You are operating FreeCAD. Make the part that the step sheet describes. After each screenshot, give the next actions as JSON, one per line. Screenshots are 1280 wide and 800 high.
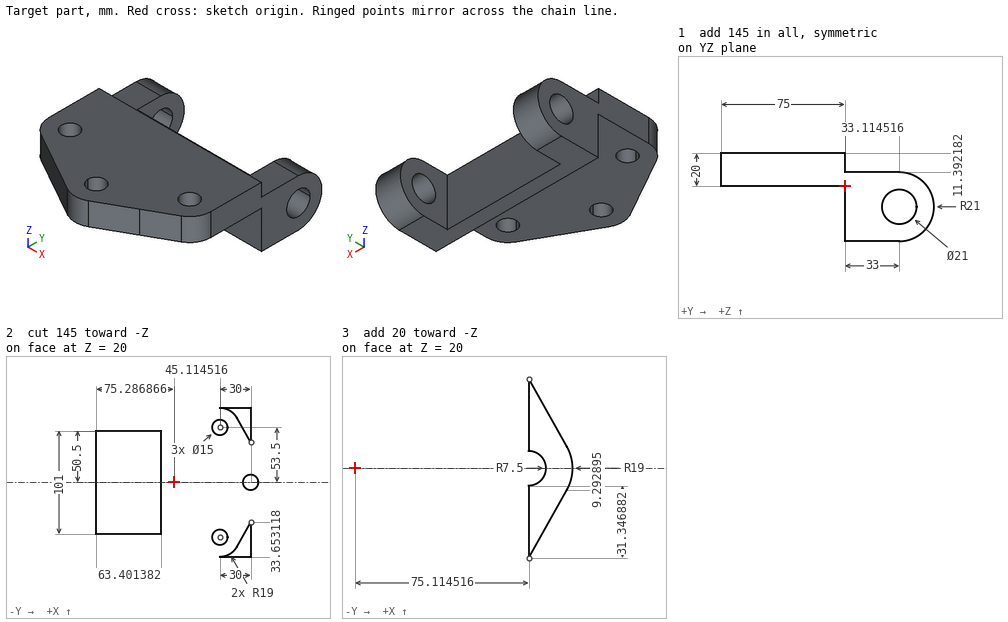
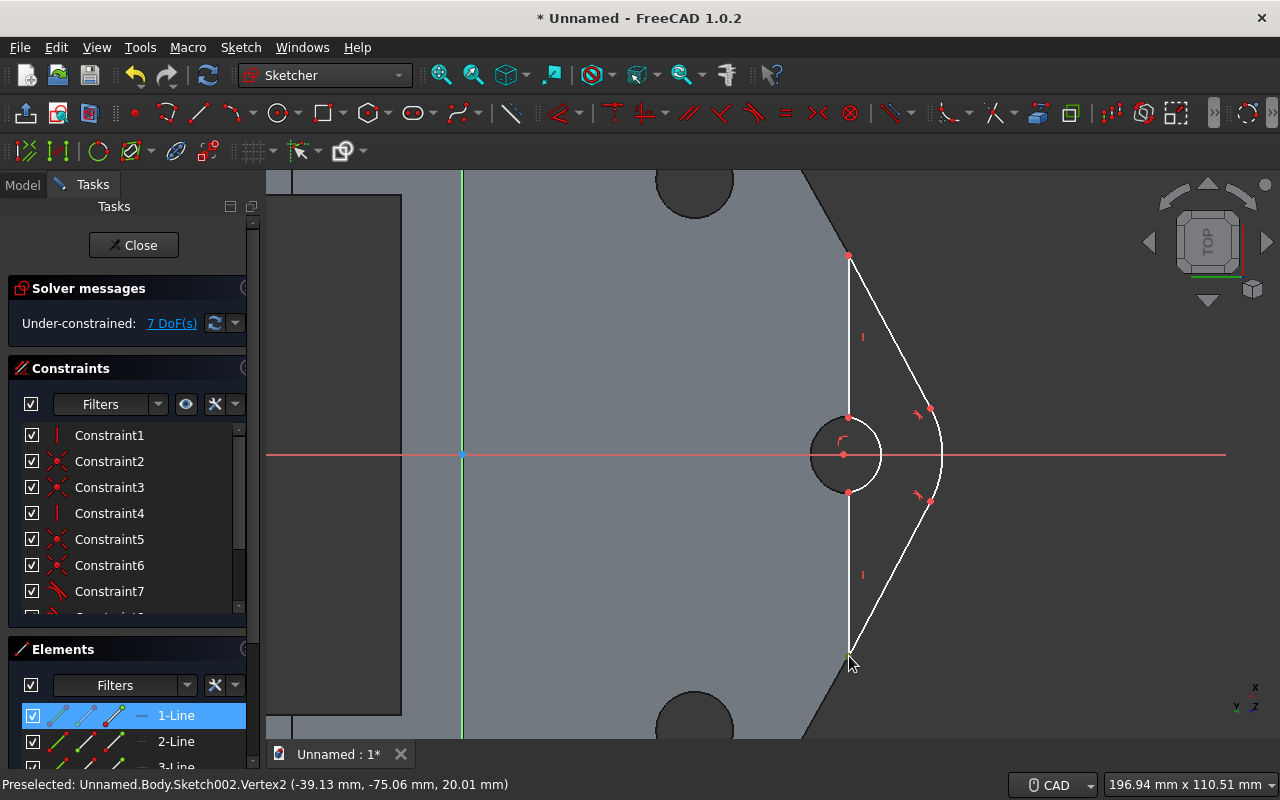
{"action": "left_click", "coordinate": [849, 255]}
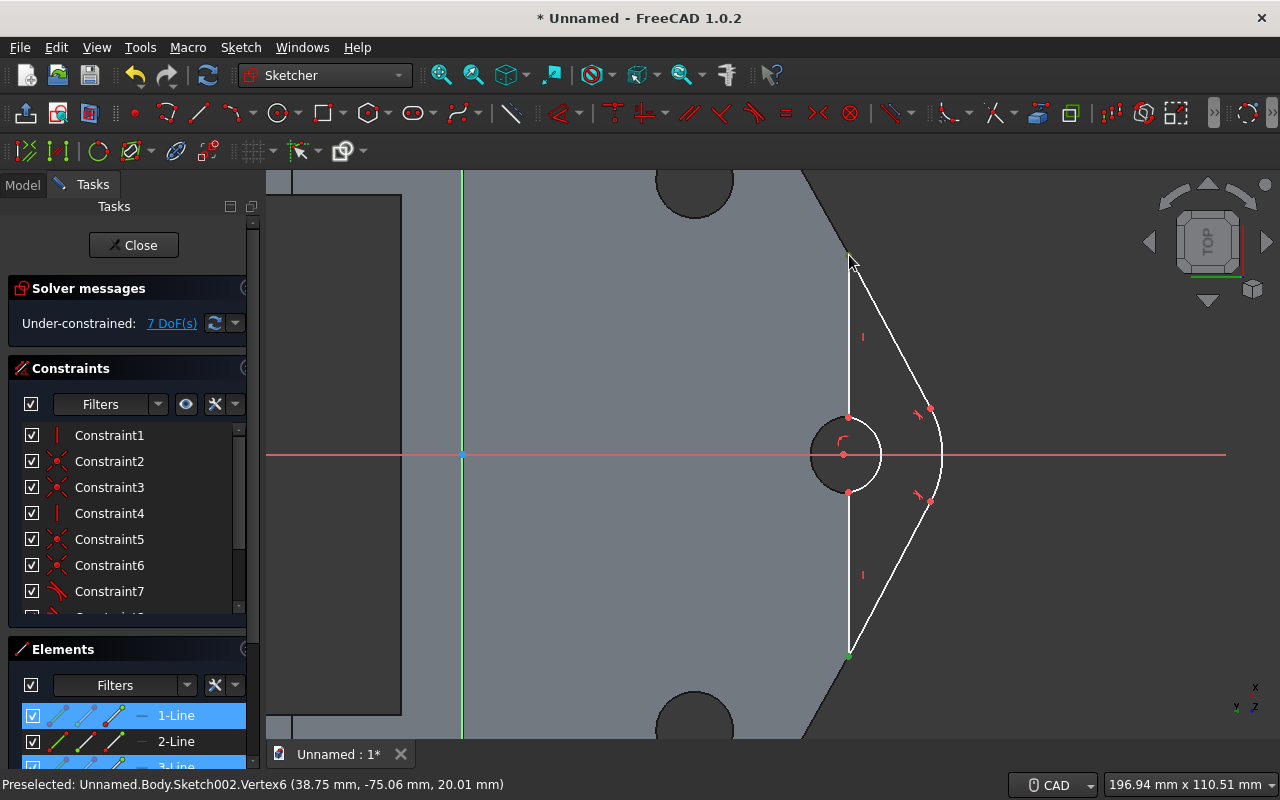
{"action": "left_click", "coordinate": [353, 455]}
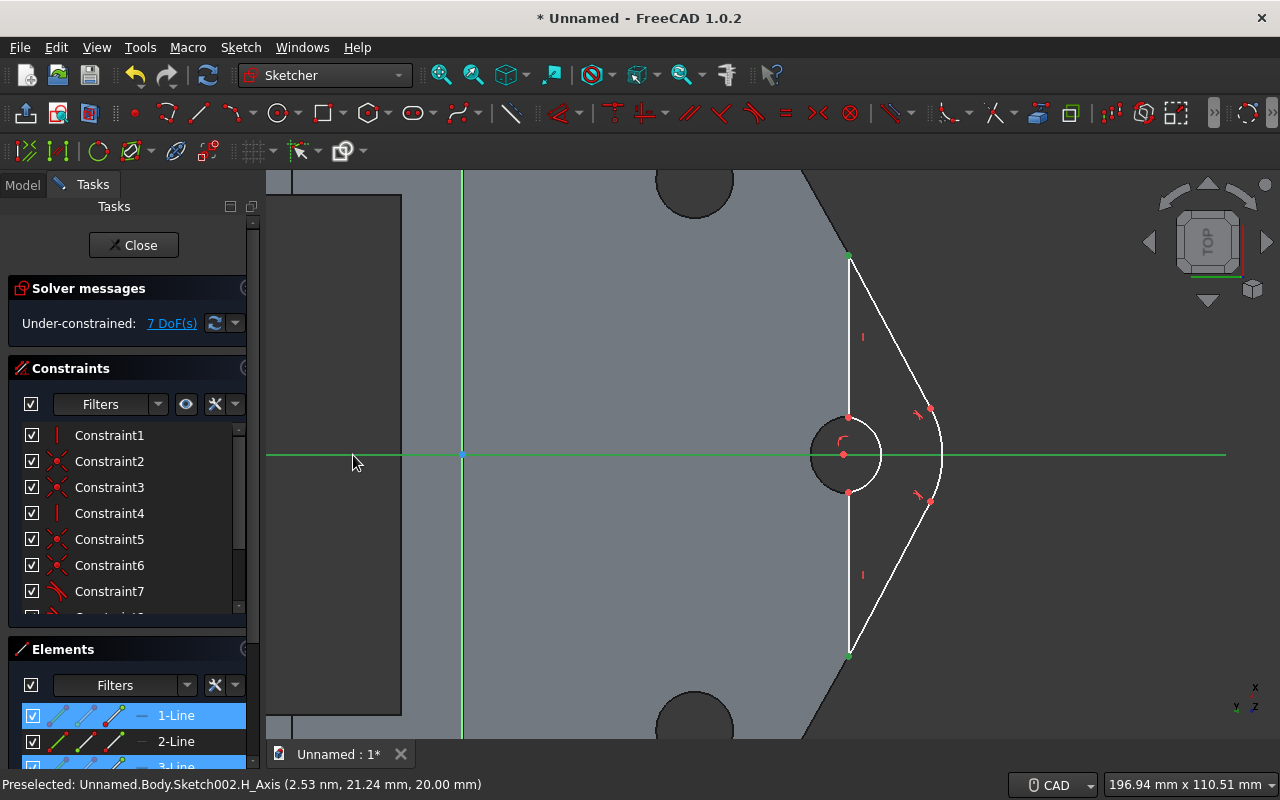
{"action": "left_click", "coordinate": [818, 114]}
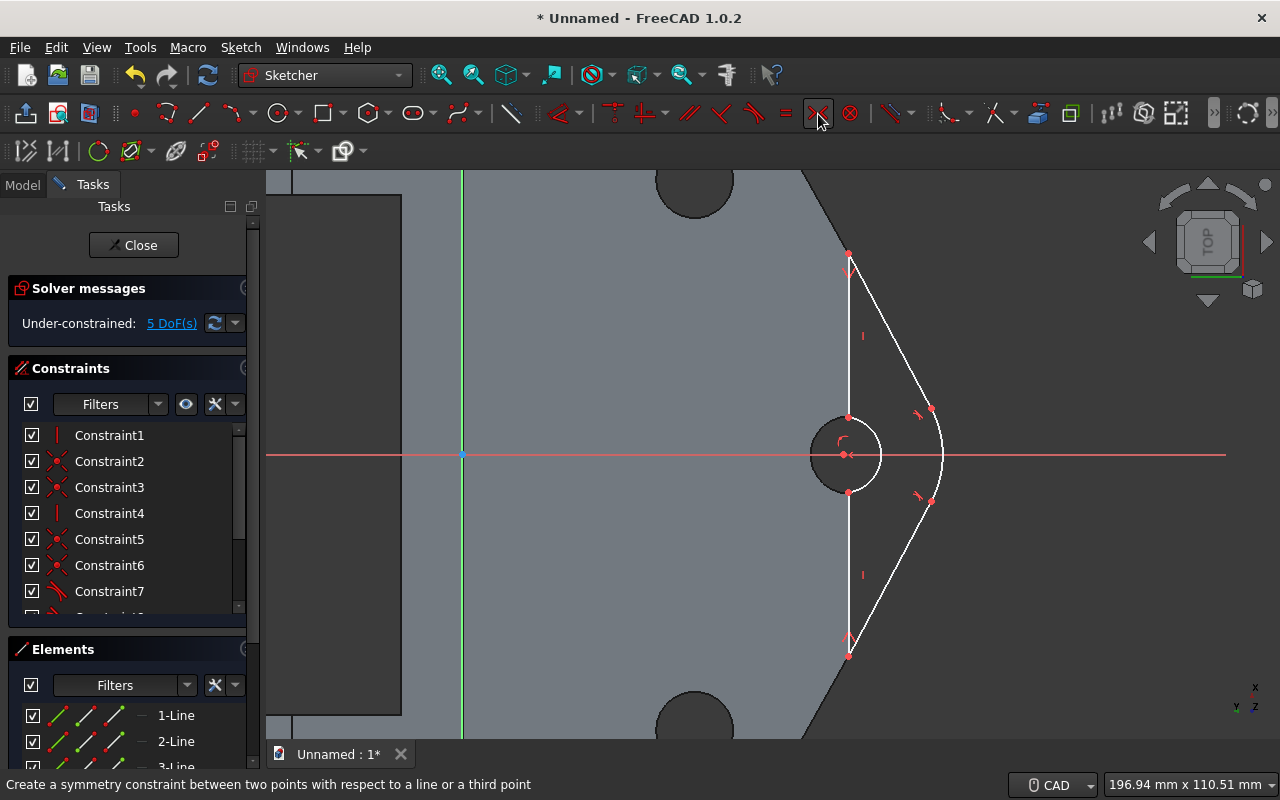
{"action": "left_click", "coordinate": [558, 114]}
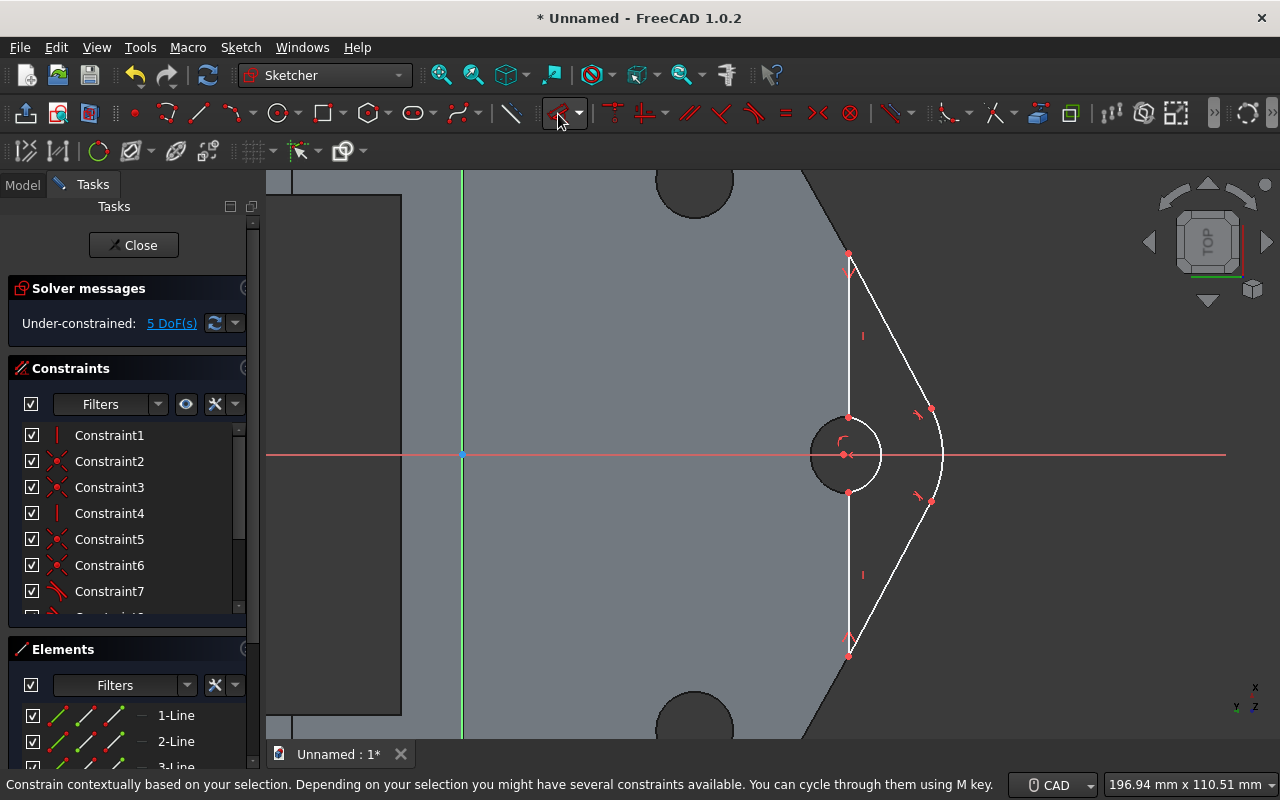
{"action": "left_click", "coordinate": [941, 474]}
{"action": "left_click", "coordinate": [972, 480]}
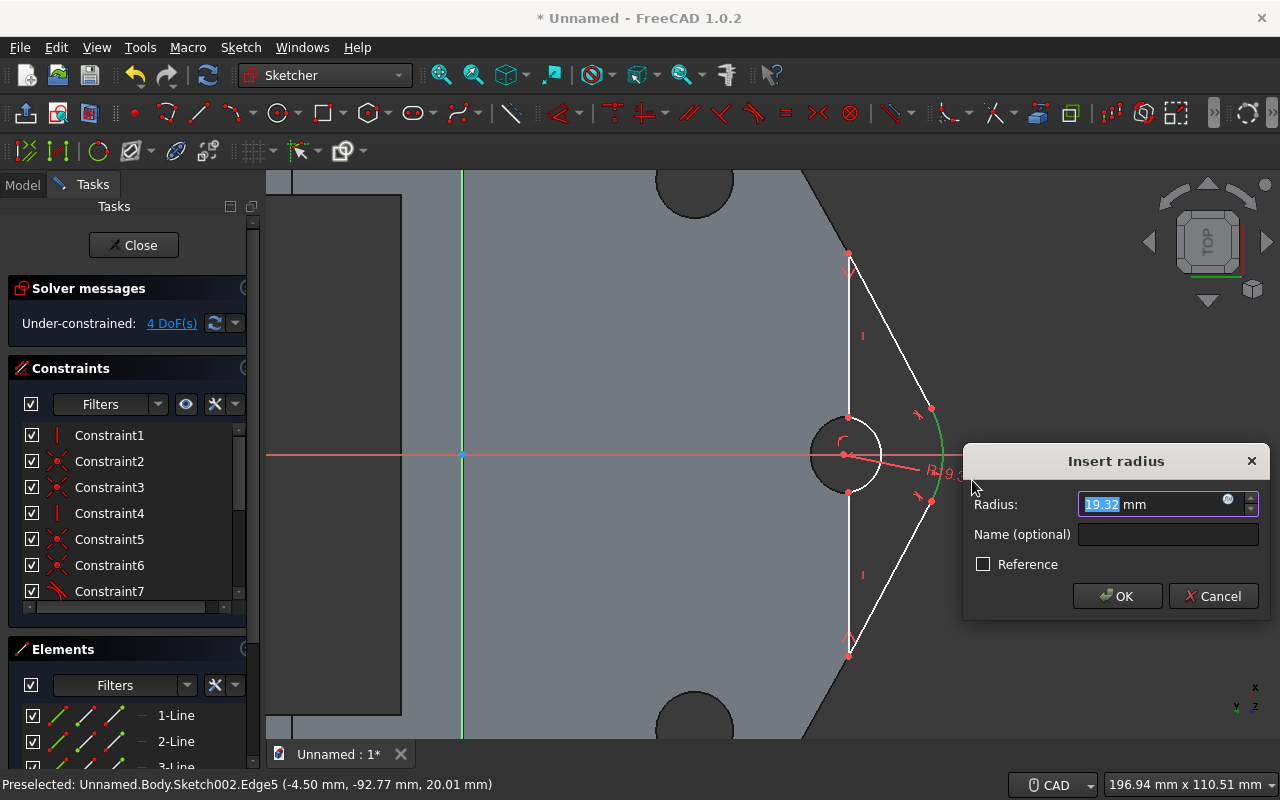
{"action": "type", "text": "19"}
{"action": "key", "text": "Return"}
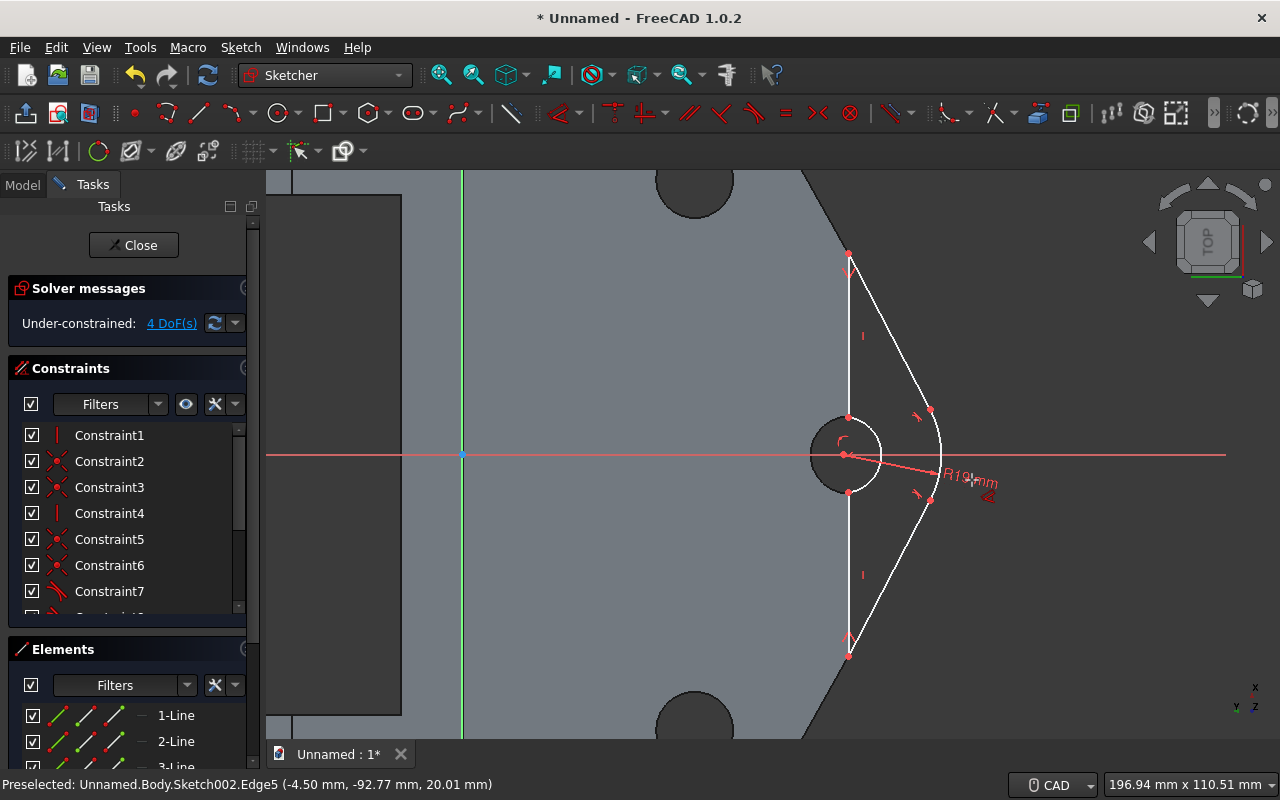
{"action": "left_click", "coordinate": [875, 475]}
{"action": "left_click", "coordinate": [902, 492]}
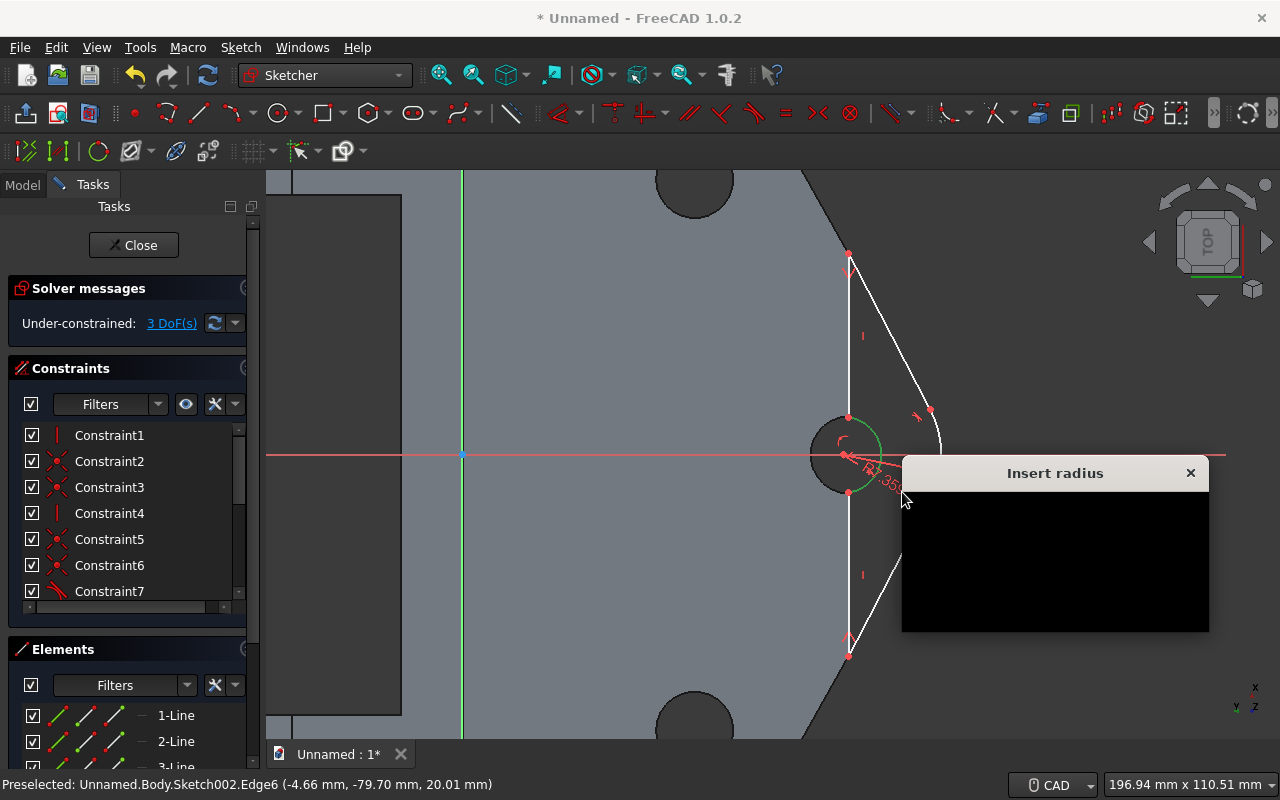
{"action": "type", "text": "7.5"}
{"action": "key", "text": "Return"}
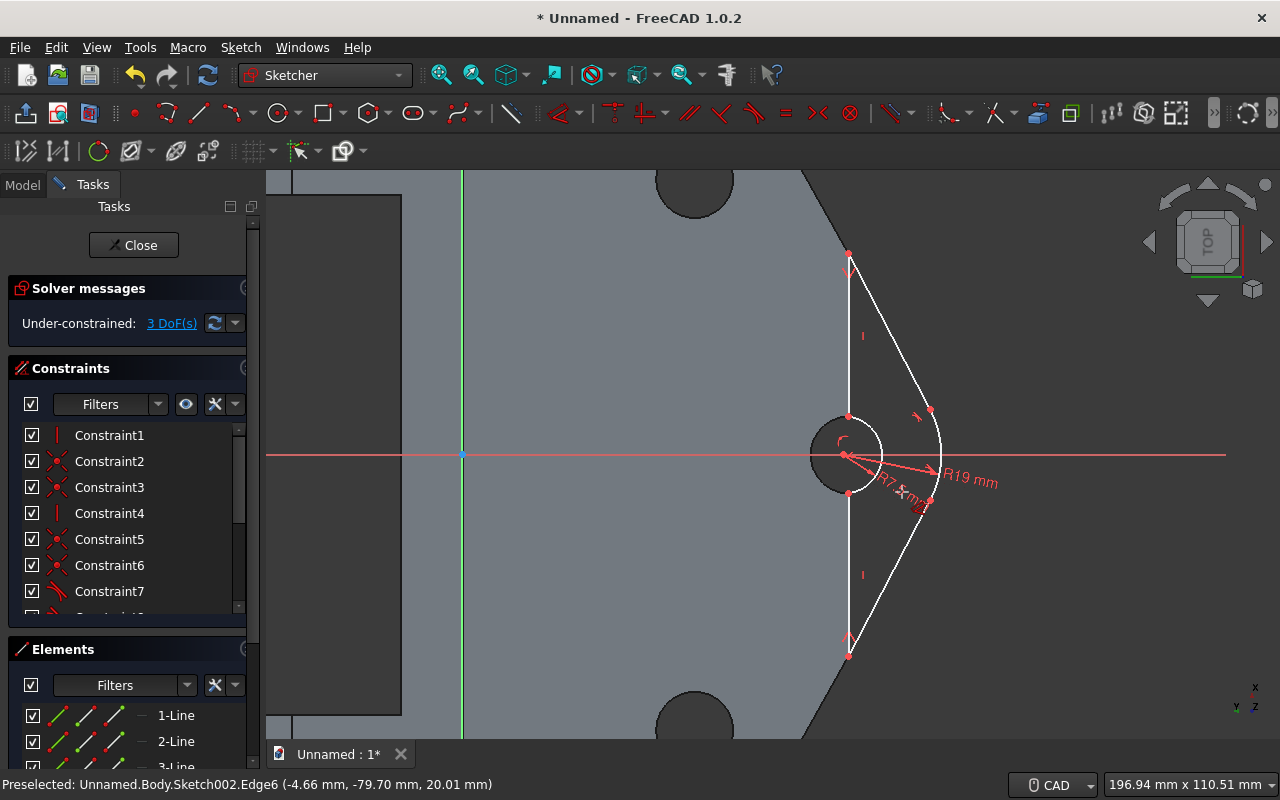
{"action": "left_click", "coordinate": [849, 542]}
{"action": "left_click", "coordinate": [883, 537]}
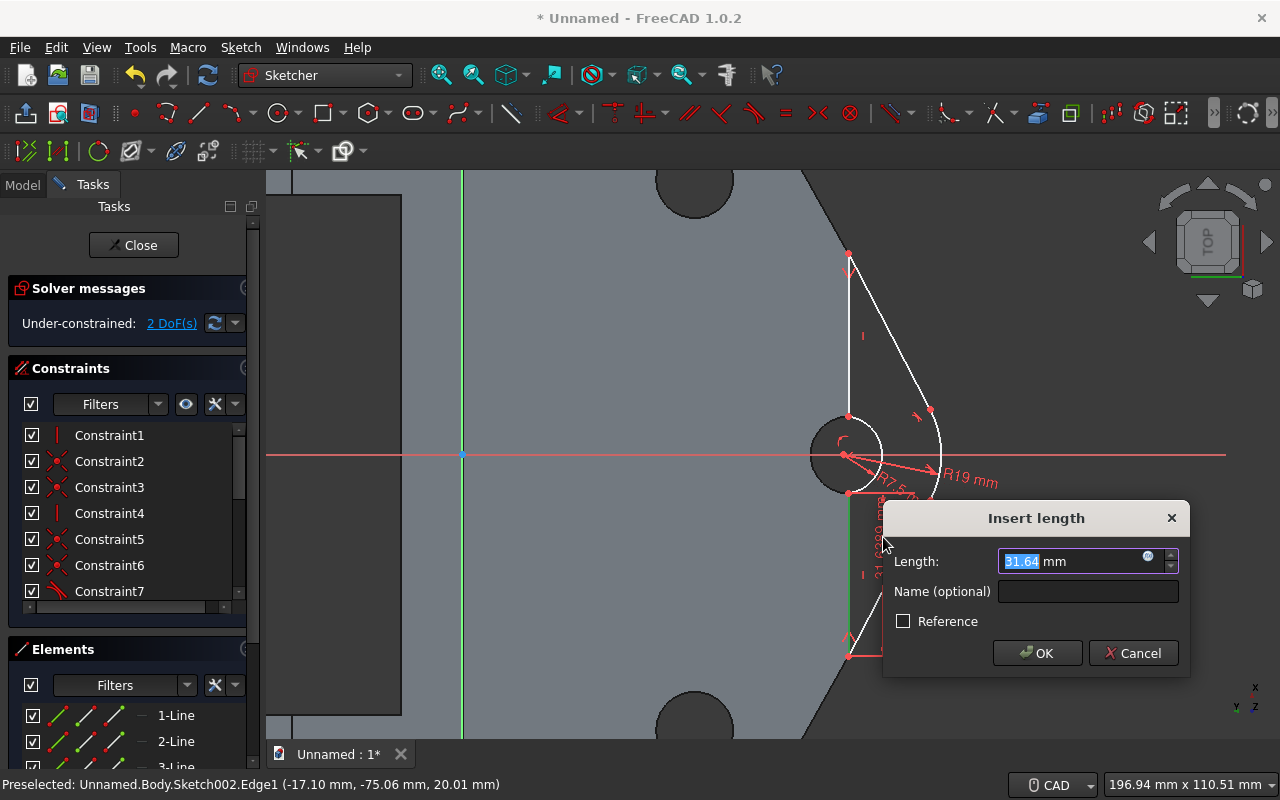
{"action": "type", "text": "31.346882"}
{"action": "key", "text": "Return"}